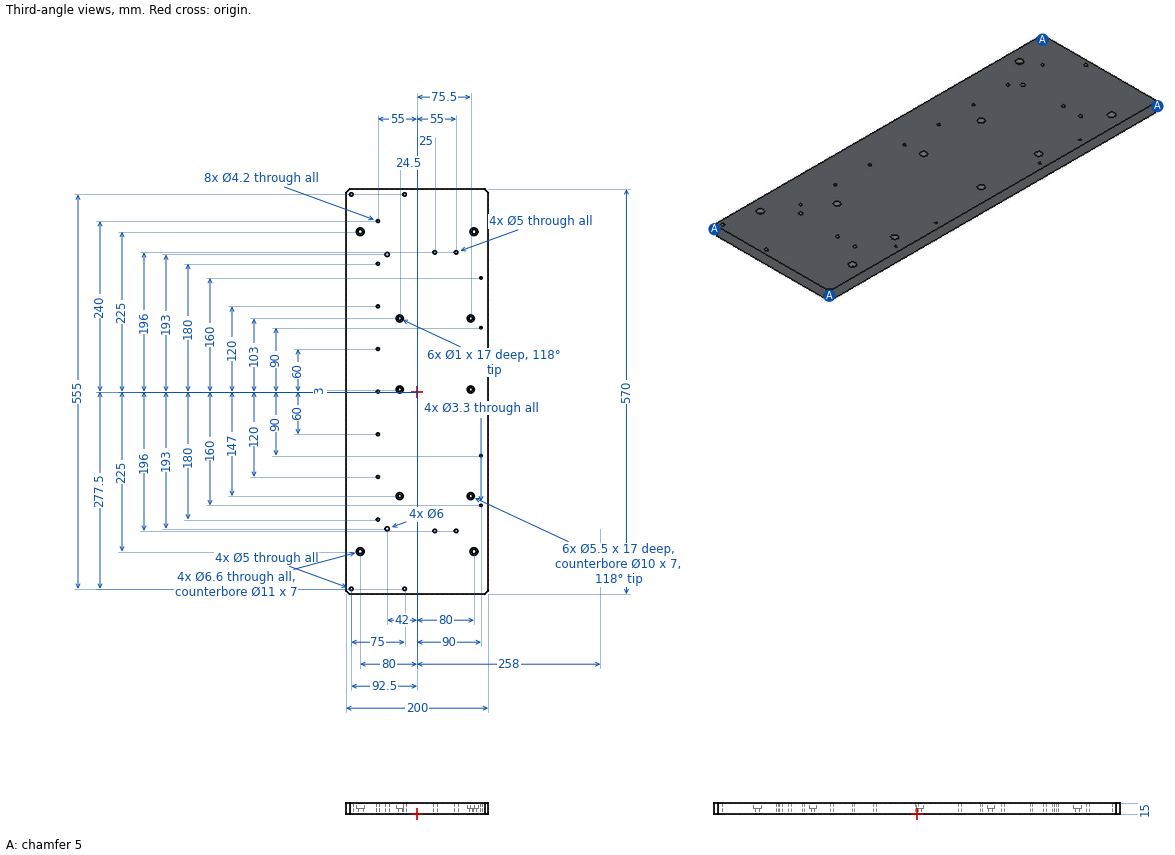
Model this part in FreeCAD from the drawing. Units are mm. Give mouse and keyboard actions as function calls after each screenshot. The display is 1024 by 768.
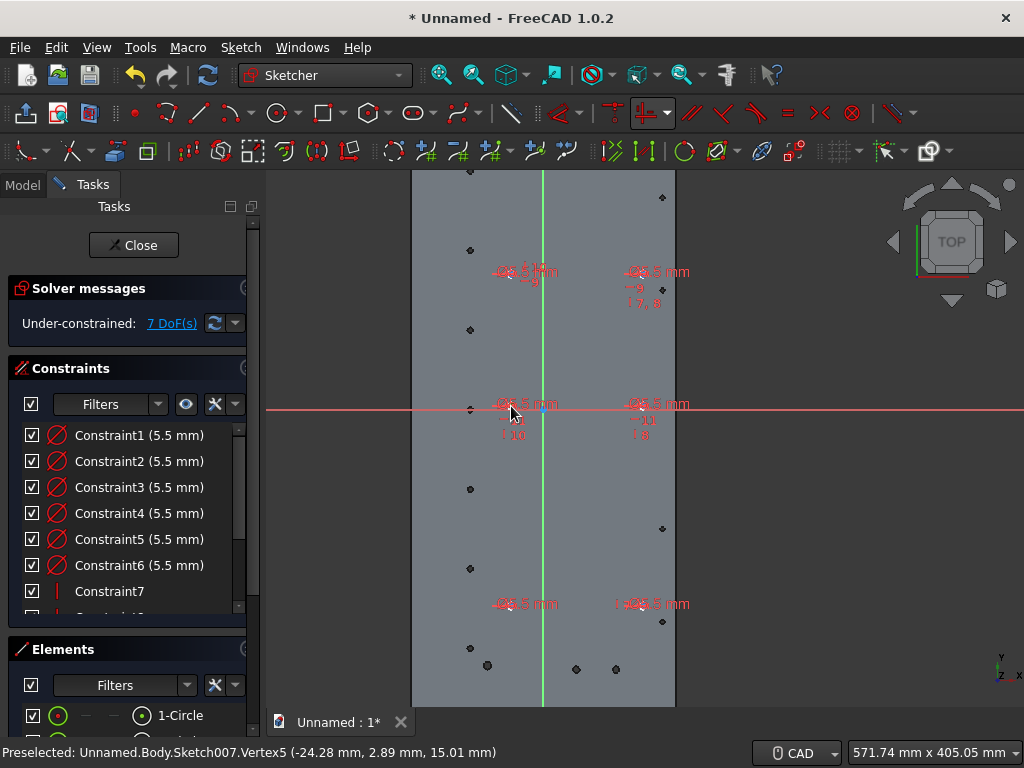
click(511, 606)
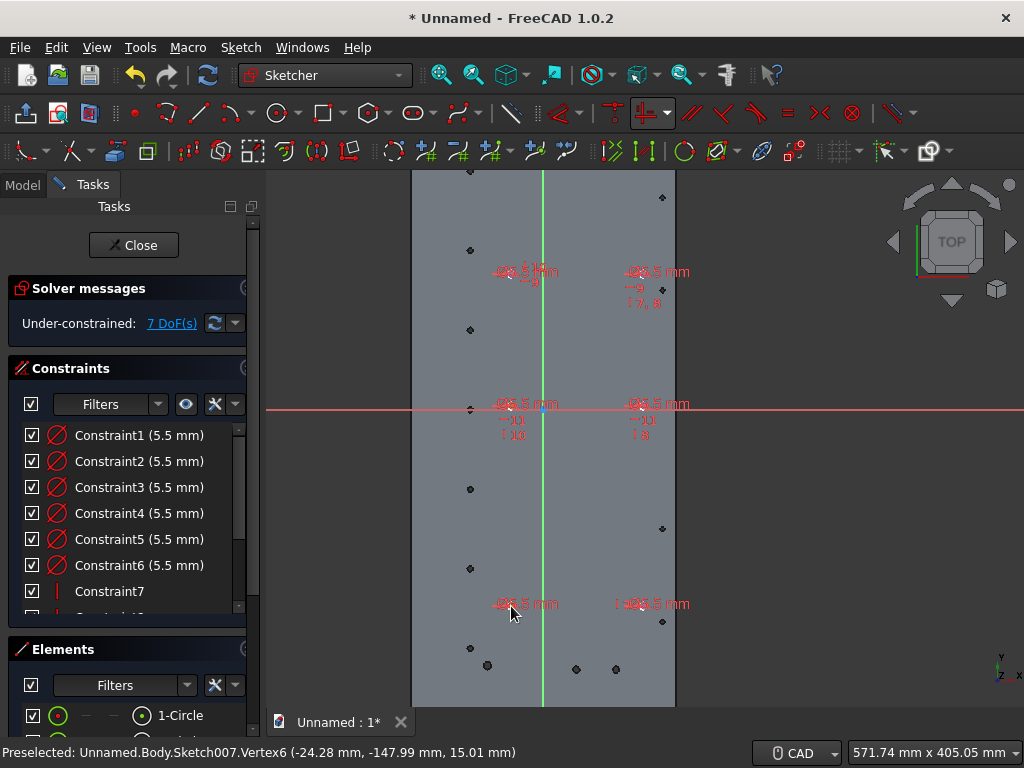
key(v)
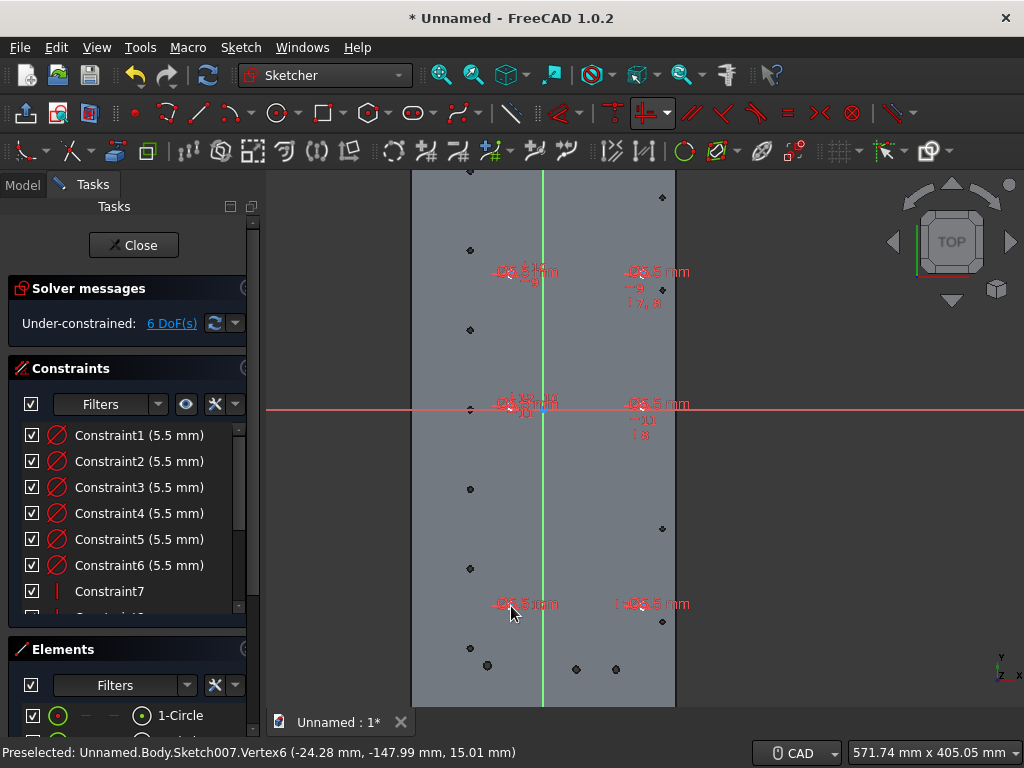
click(643, 606)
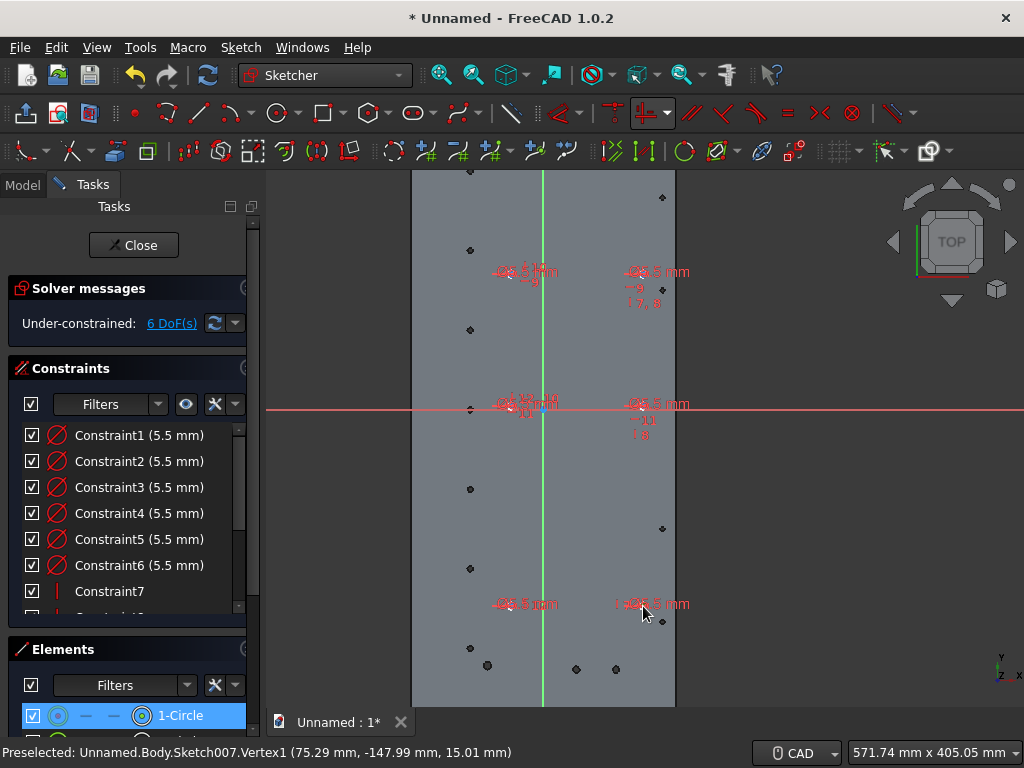
click(511, 606)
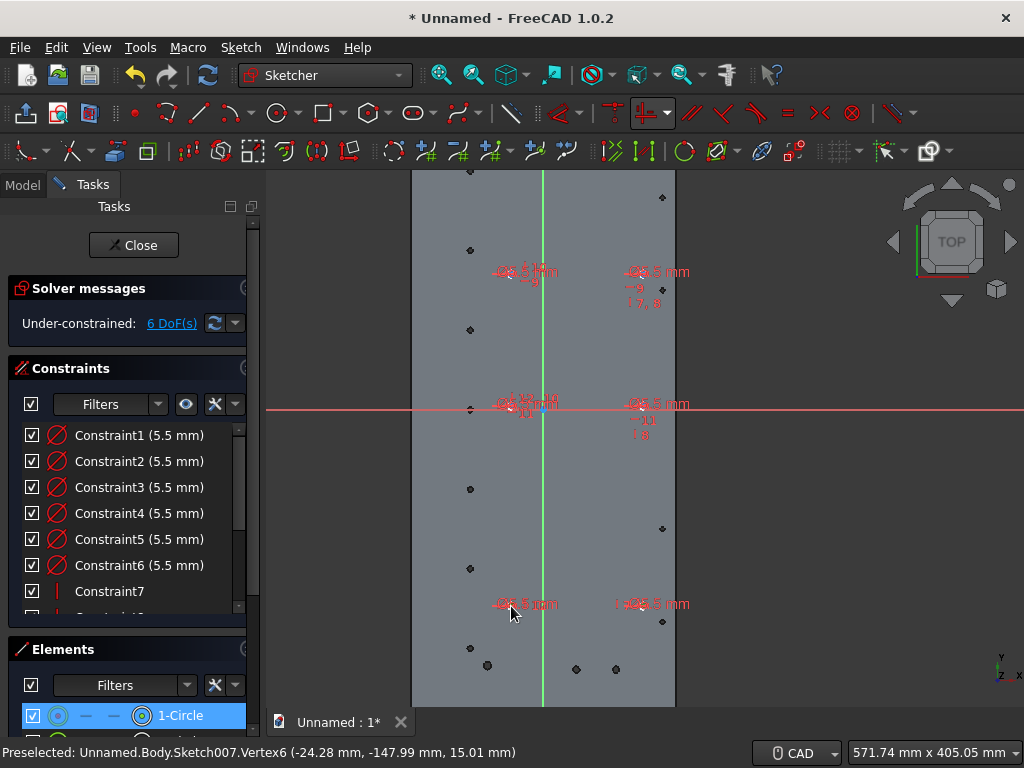
click(670, 114)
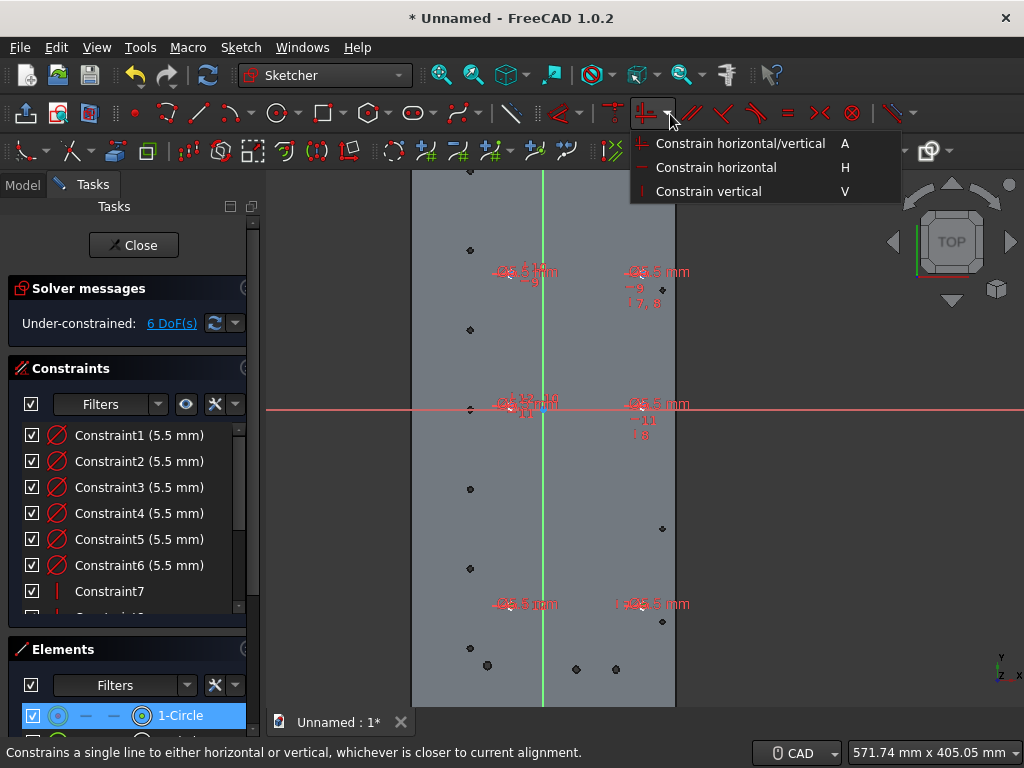
click(766, 167)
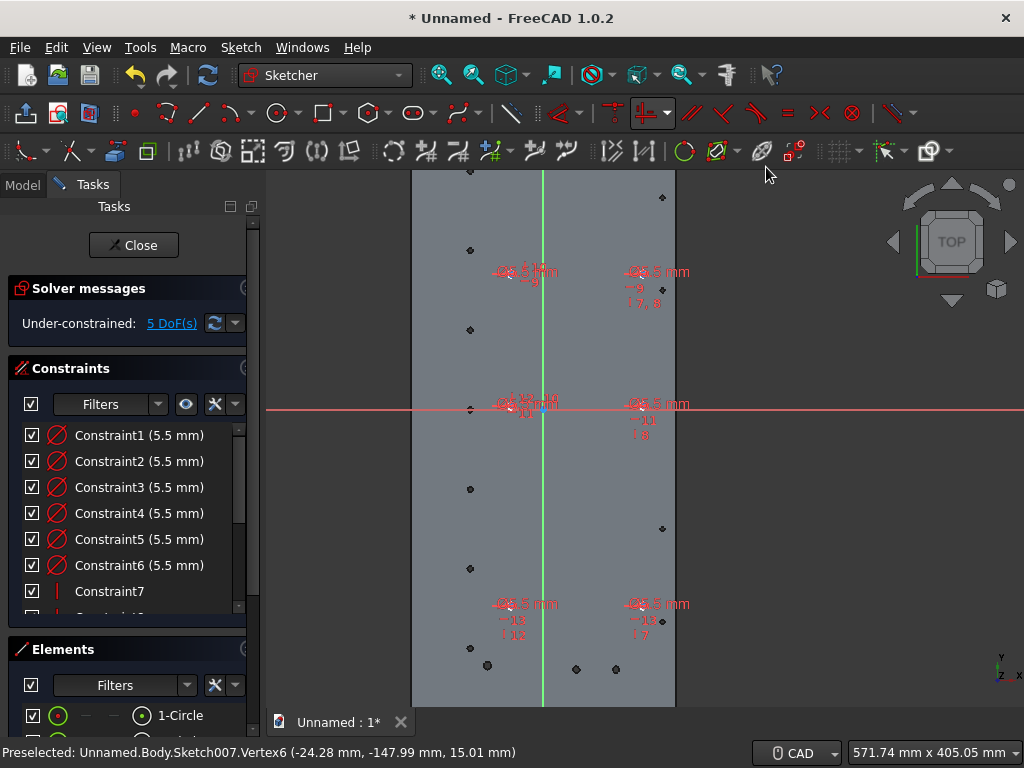
click(558, 114)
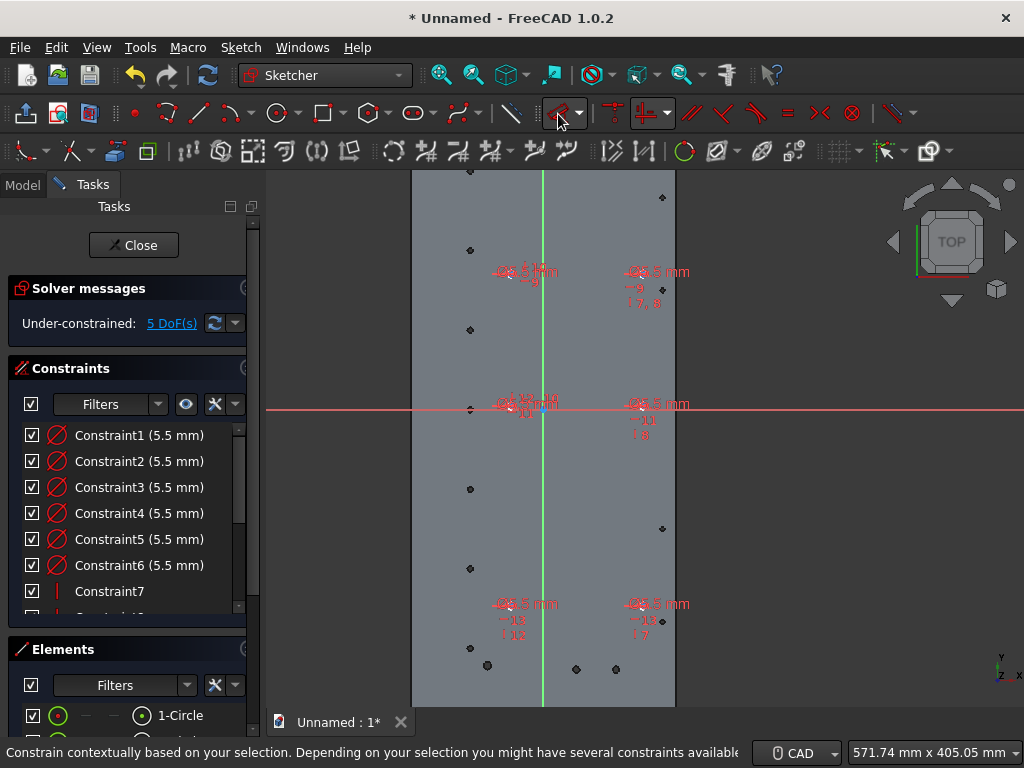
scroll(643, 406, up, 12)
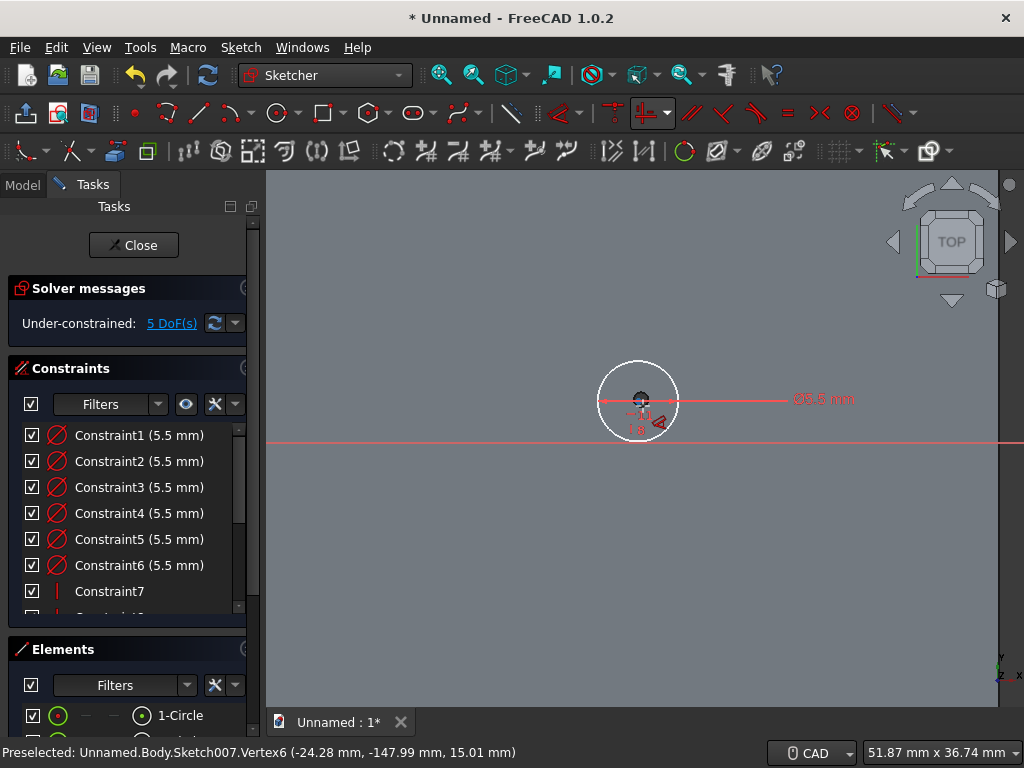
click(638, 401)
click(696, 422)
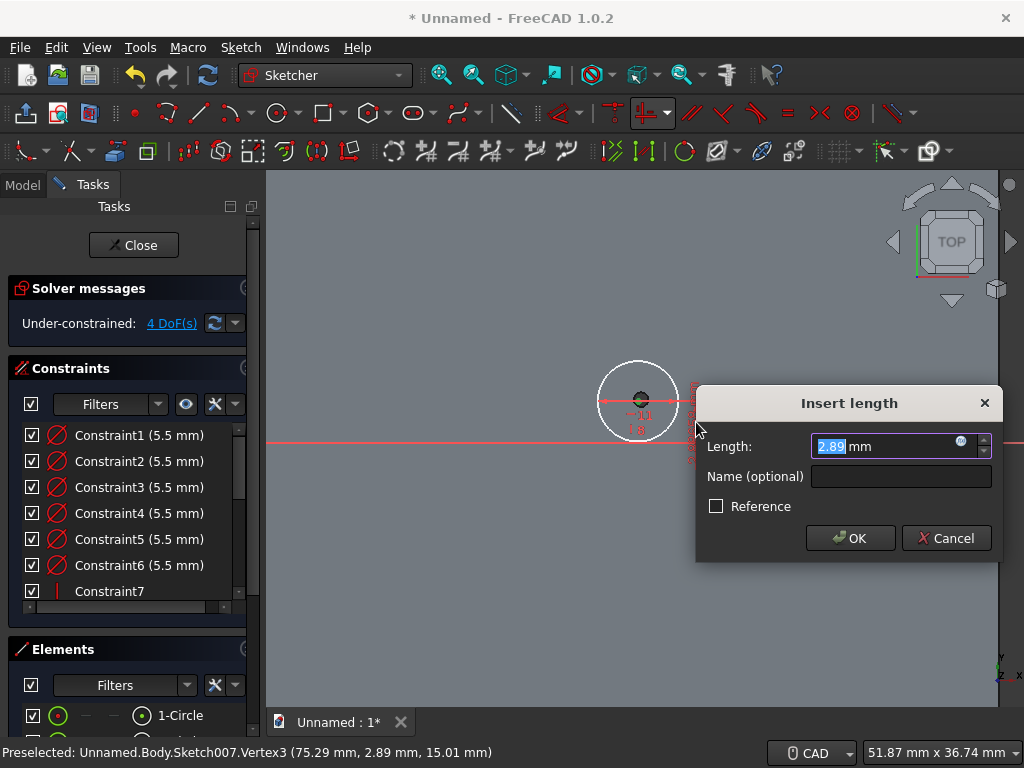
text(3)
key(Return)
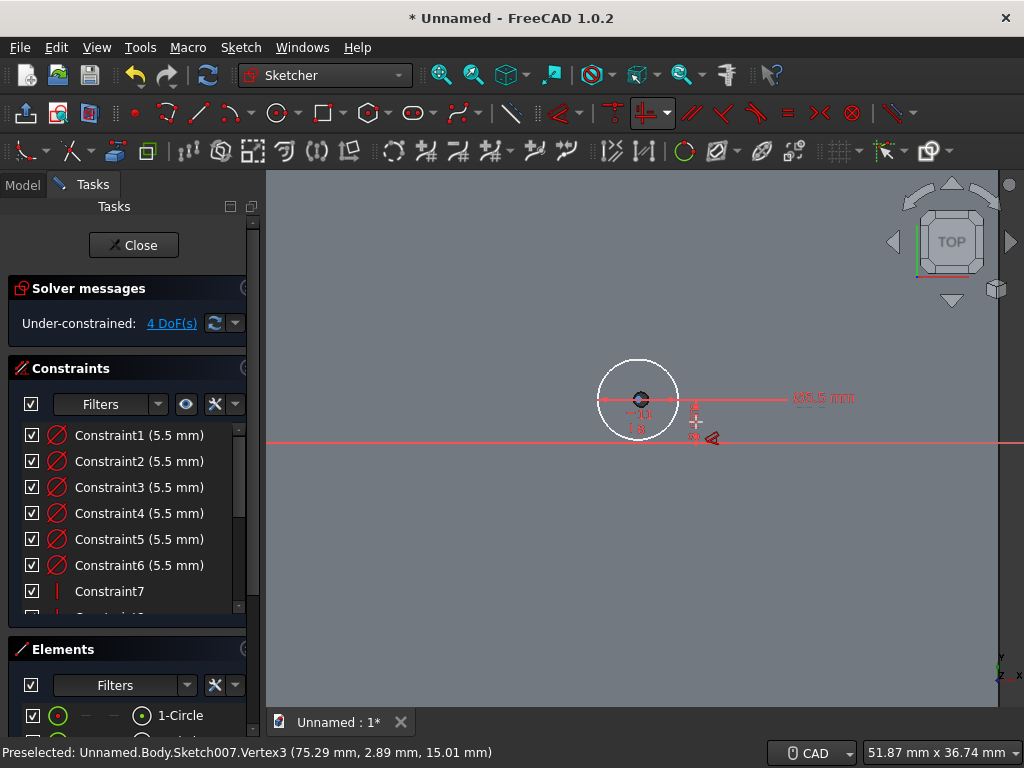
scroll(643, 406, down, 12)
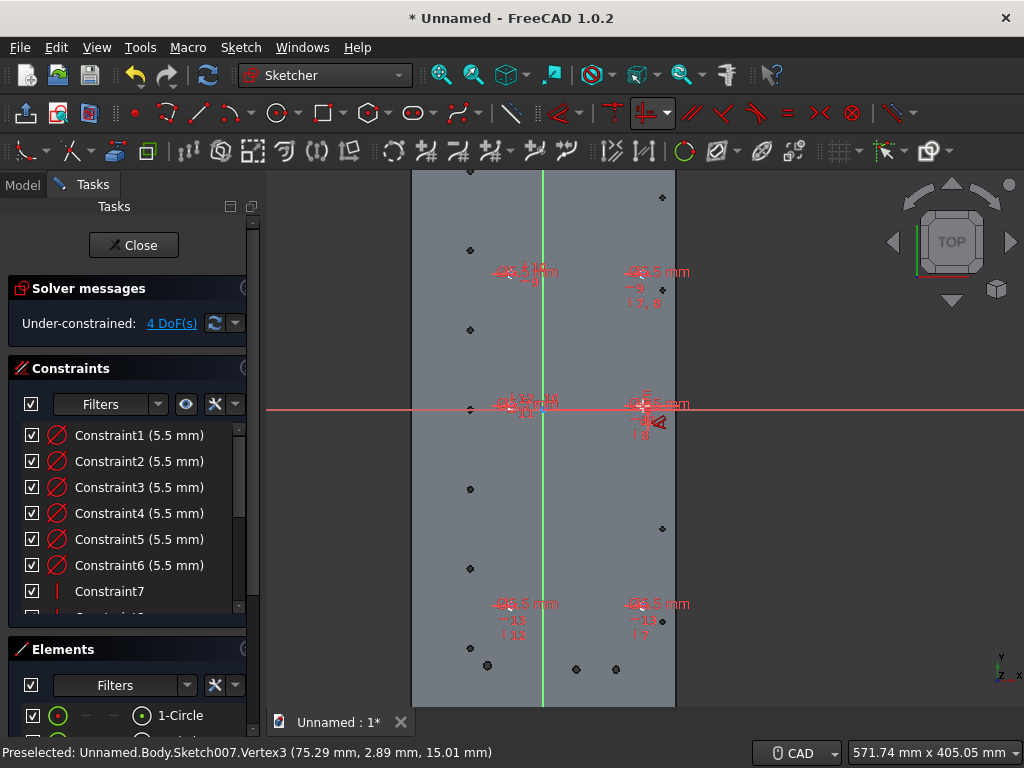
click(643, 606)
click(677, 508)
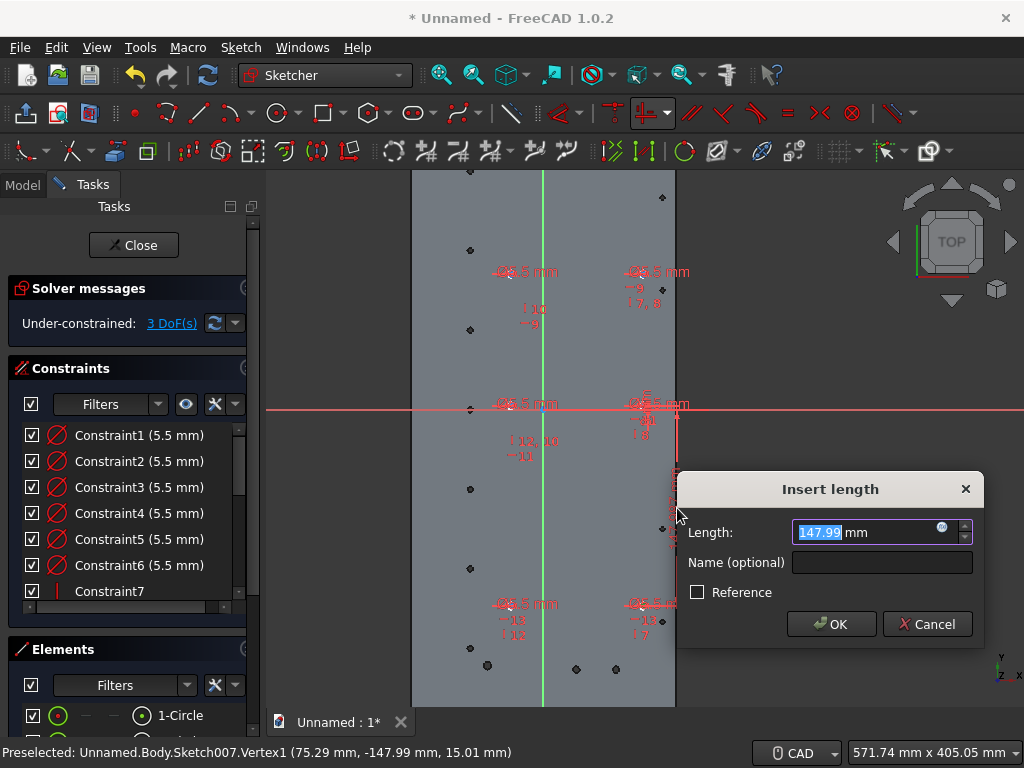
text(147)
key(Return)